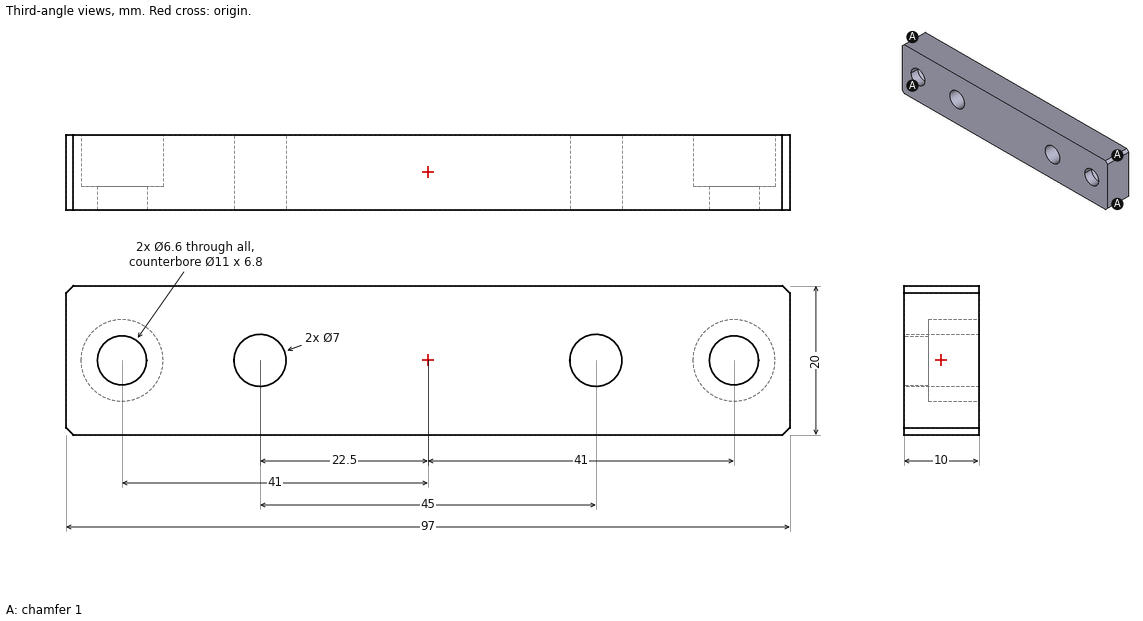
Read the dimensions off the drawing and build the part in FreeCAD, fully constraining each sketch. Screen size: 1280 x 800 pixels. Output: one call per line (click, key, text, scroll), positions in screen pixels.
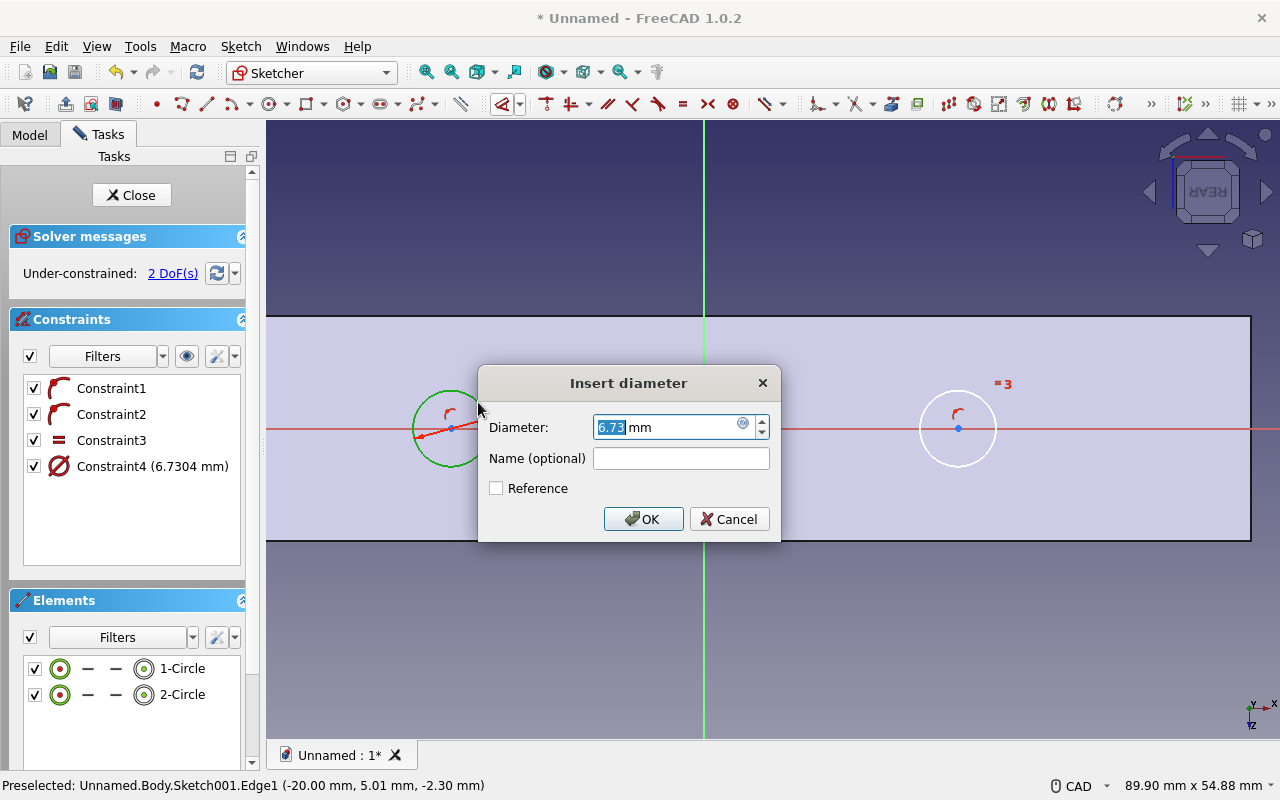
text(7)
key(Return)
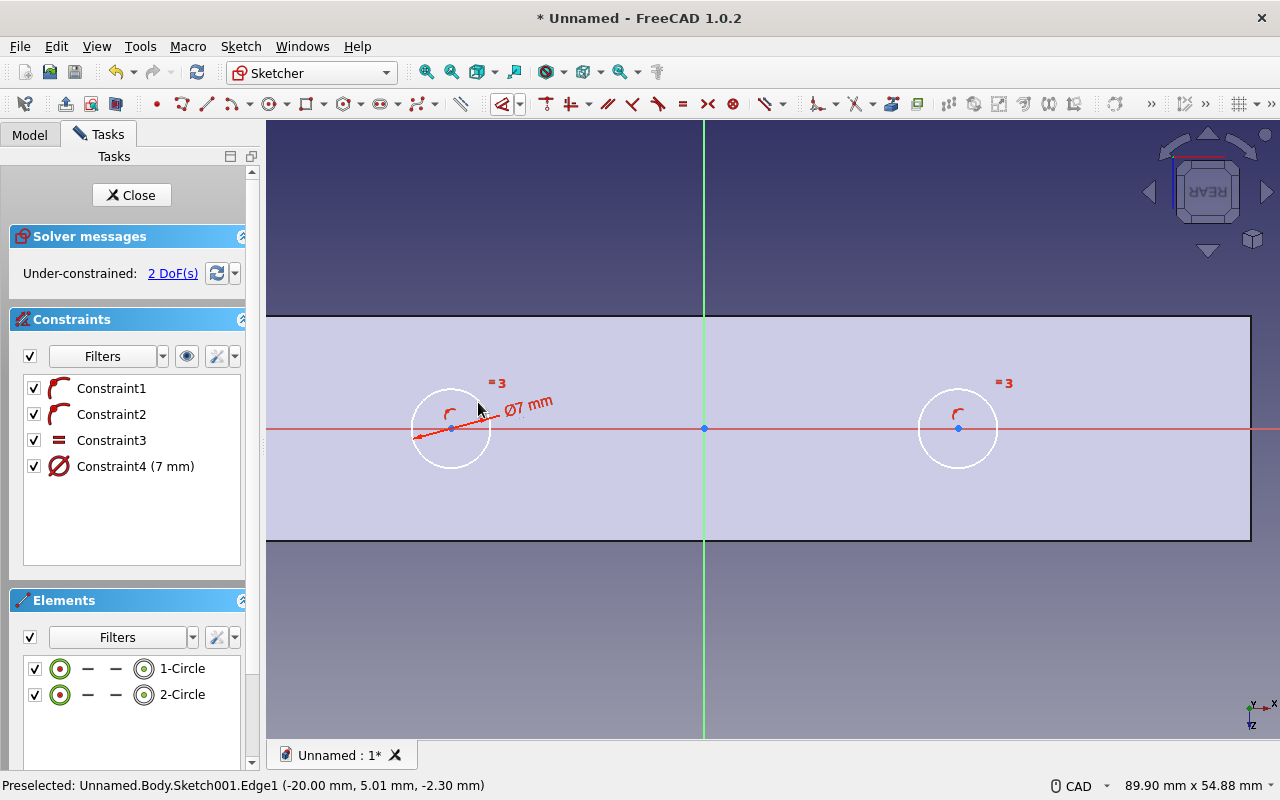
click(451, 429)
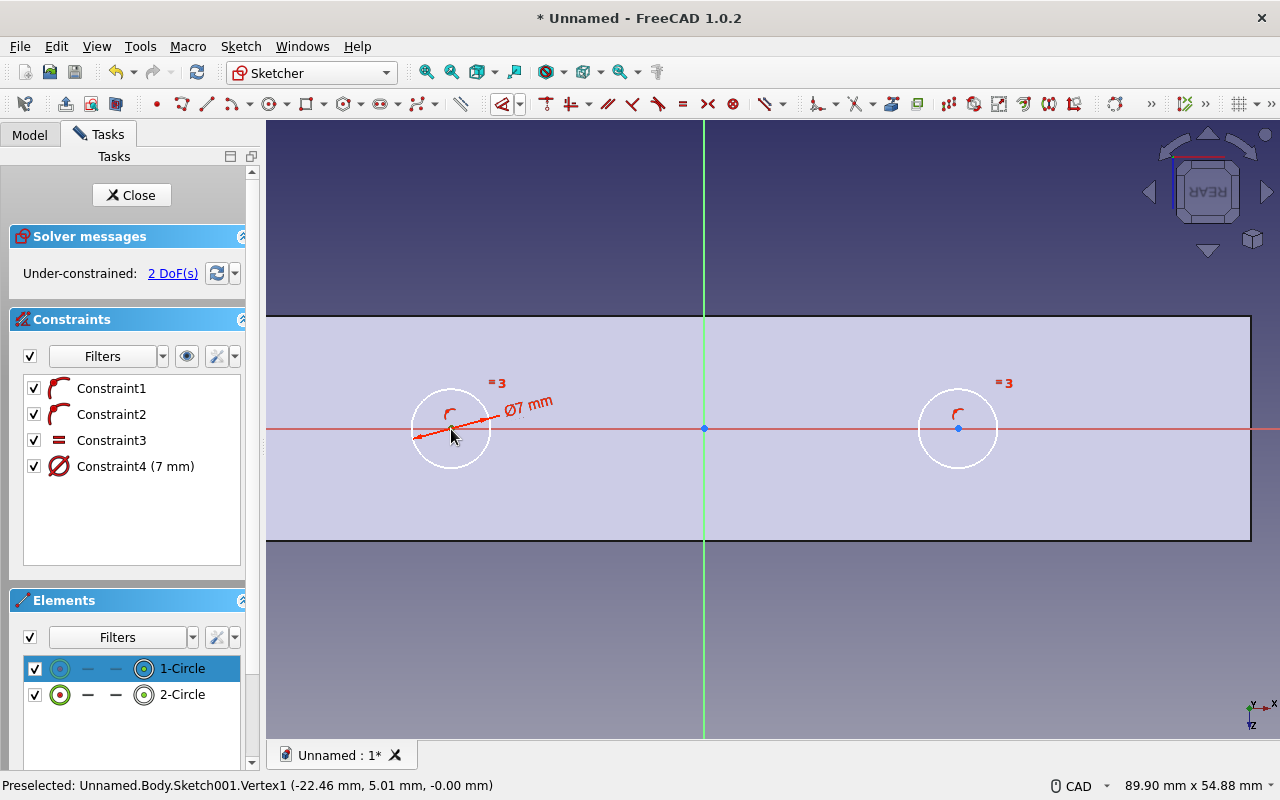
click(958, 429)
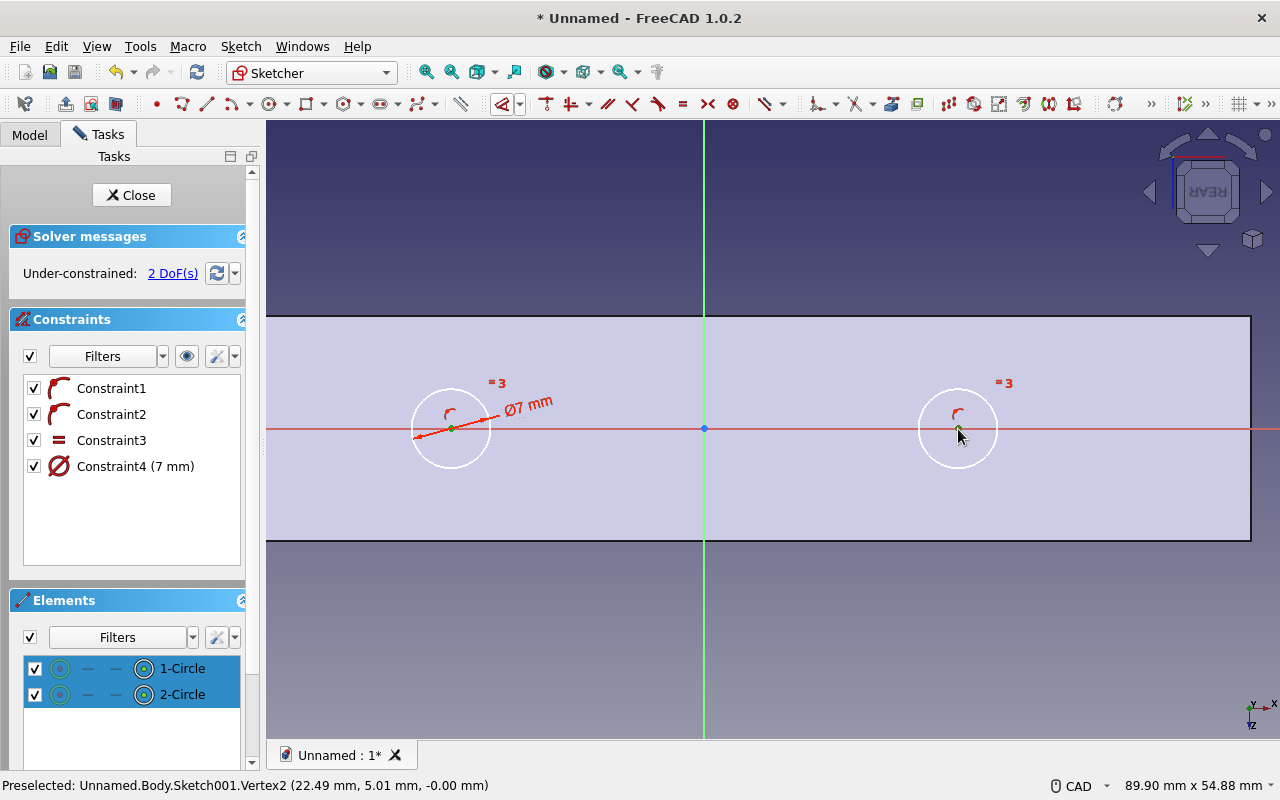
click(520, 104)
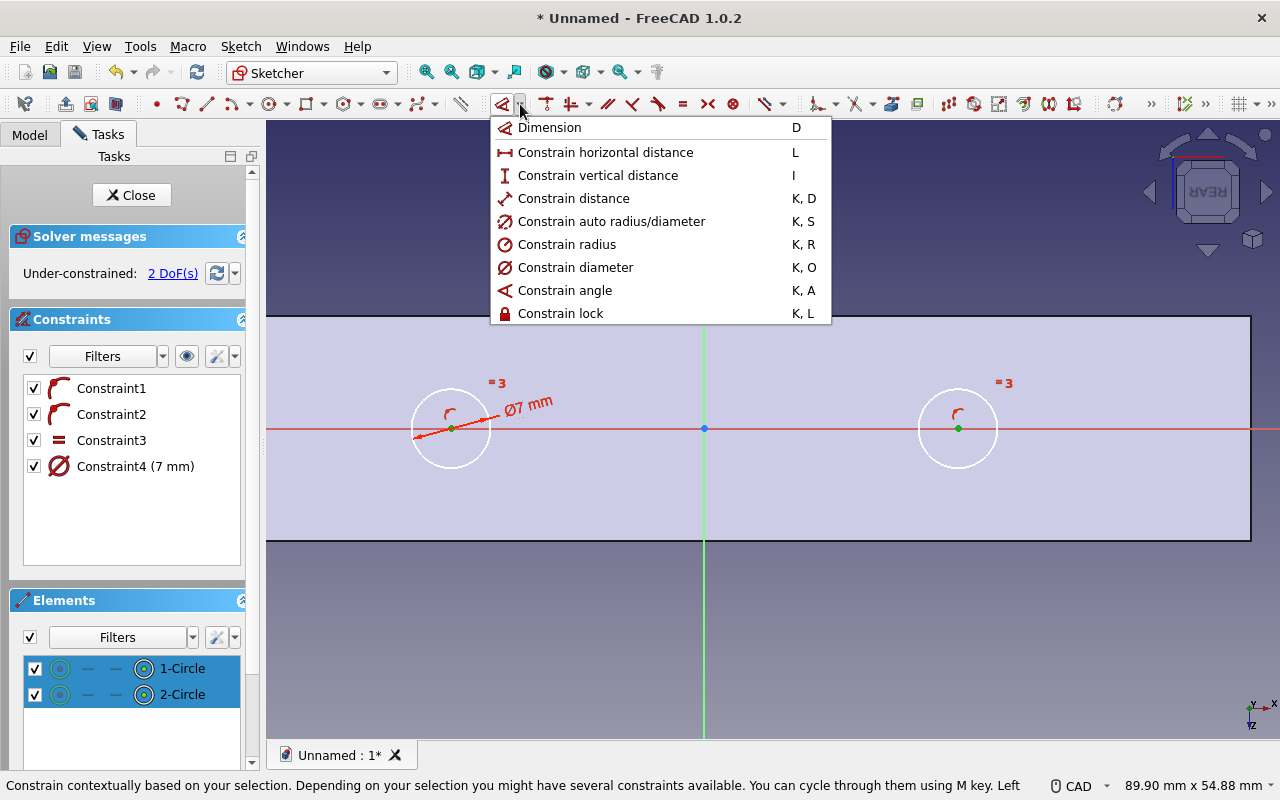
click(661, 152)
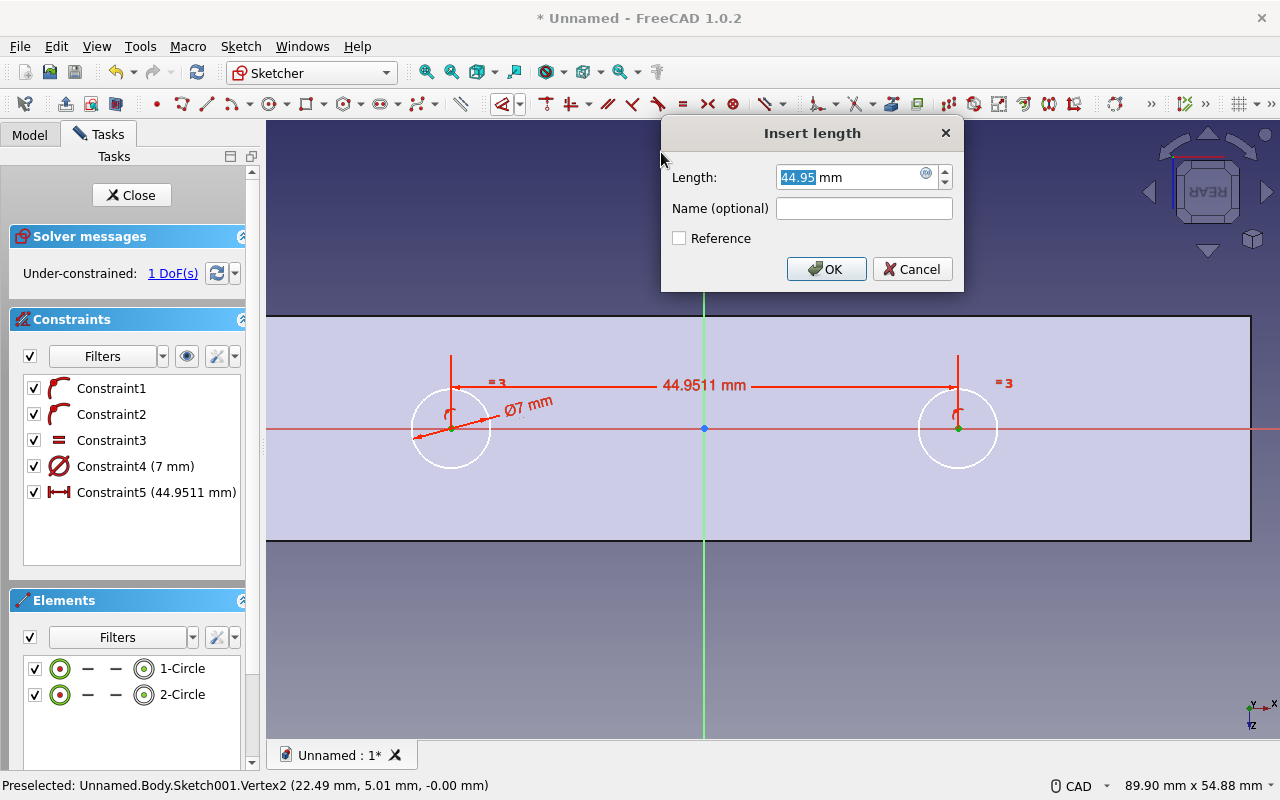
text(45)
key(Return)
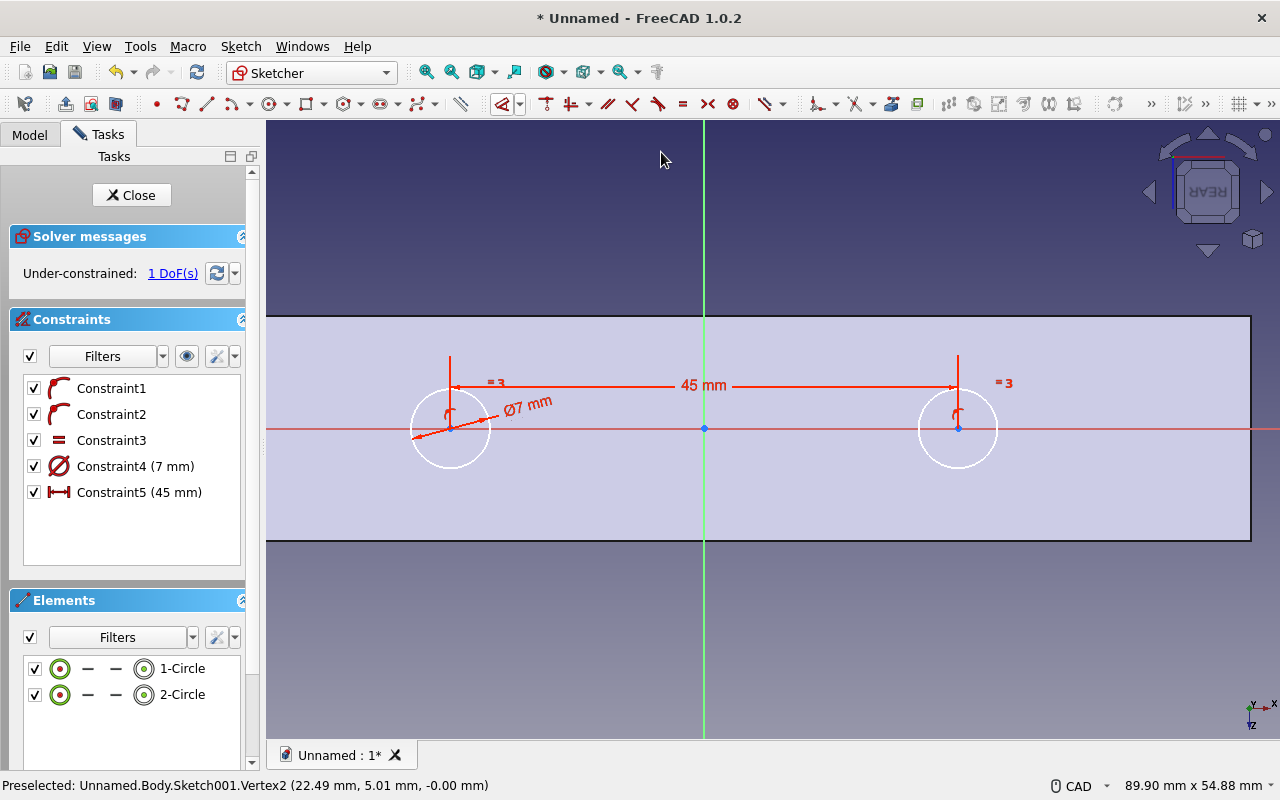
click(450, 429)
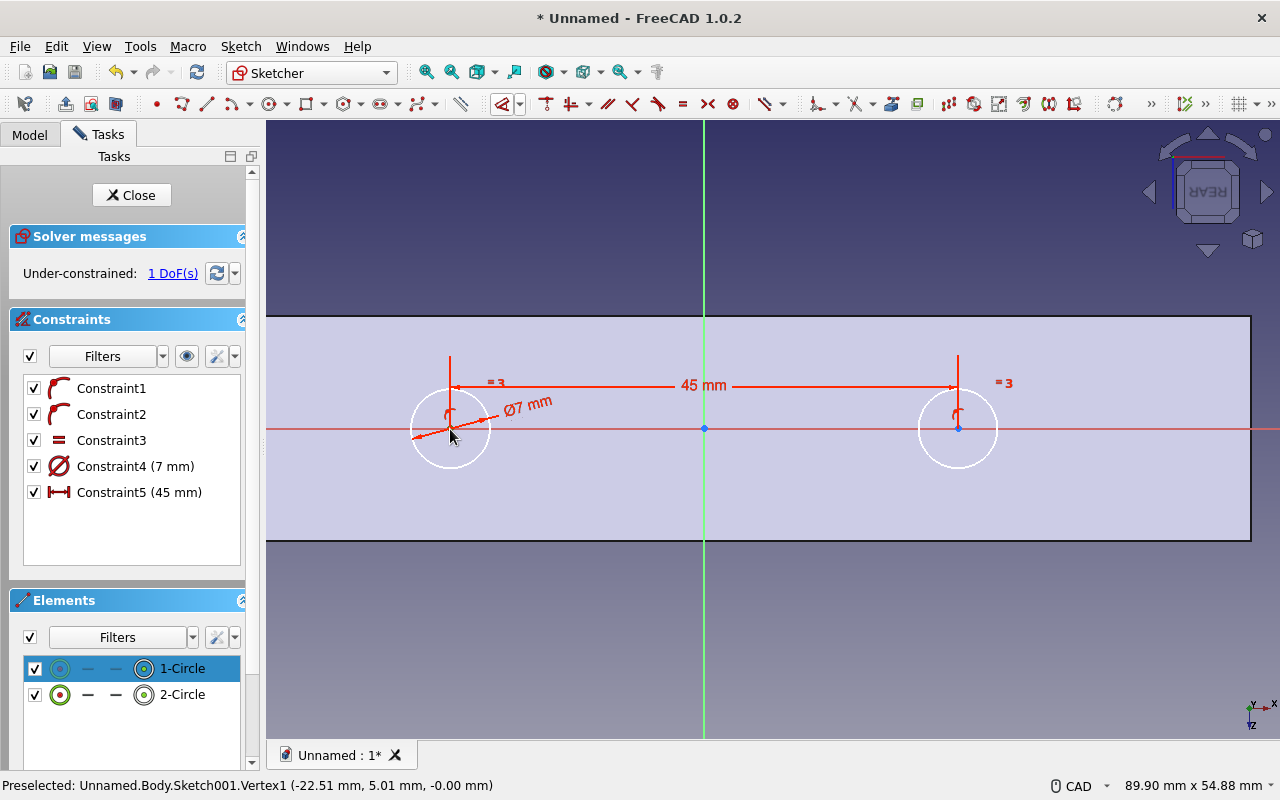
key(l)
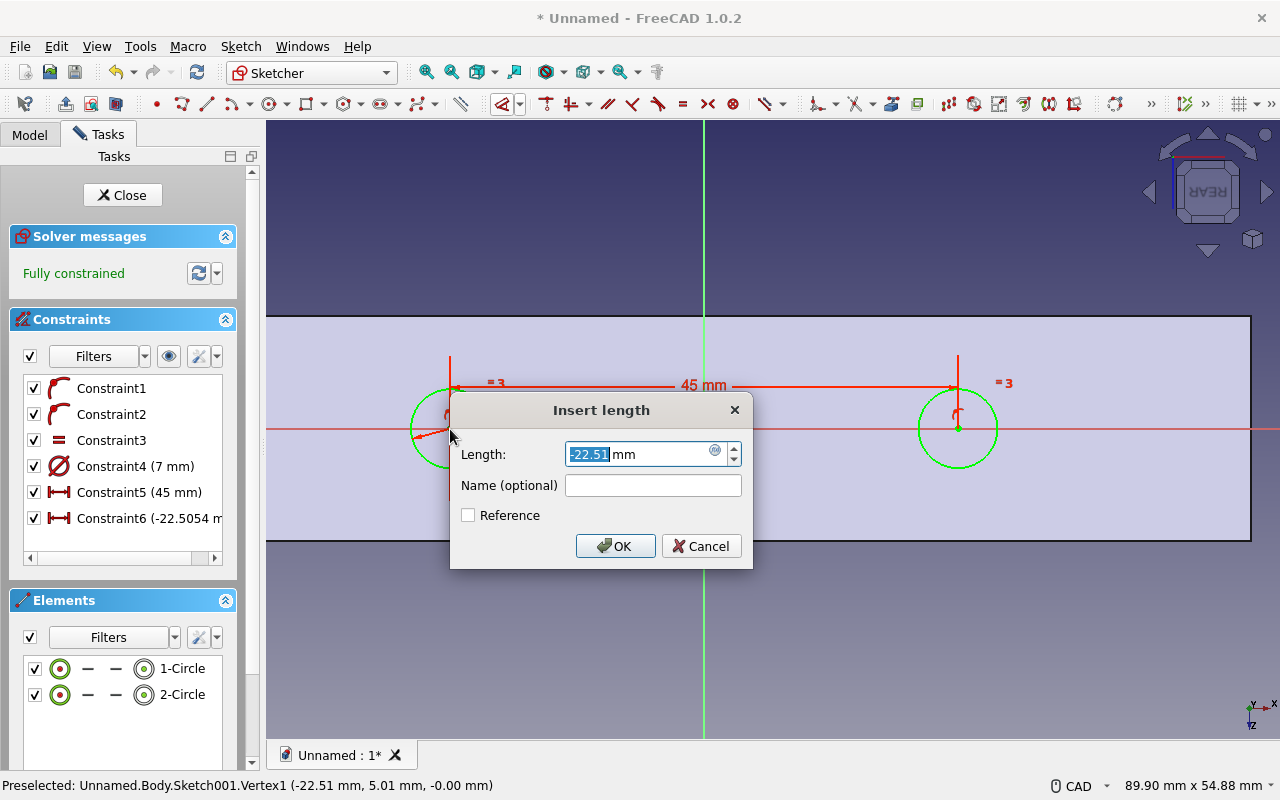
text(-22.5)
key(Return)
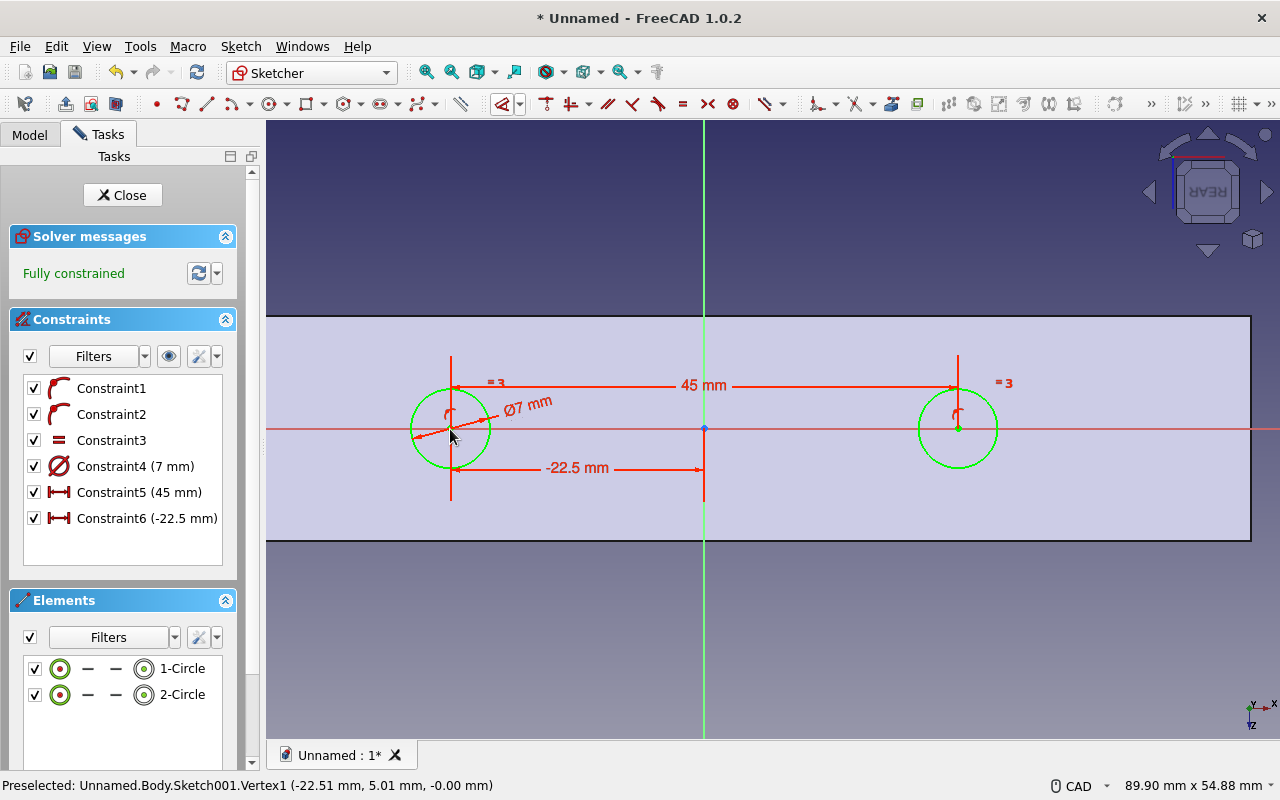
click(123, 195)